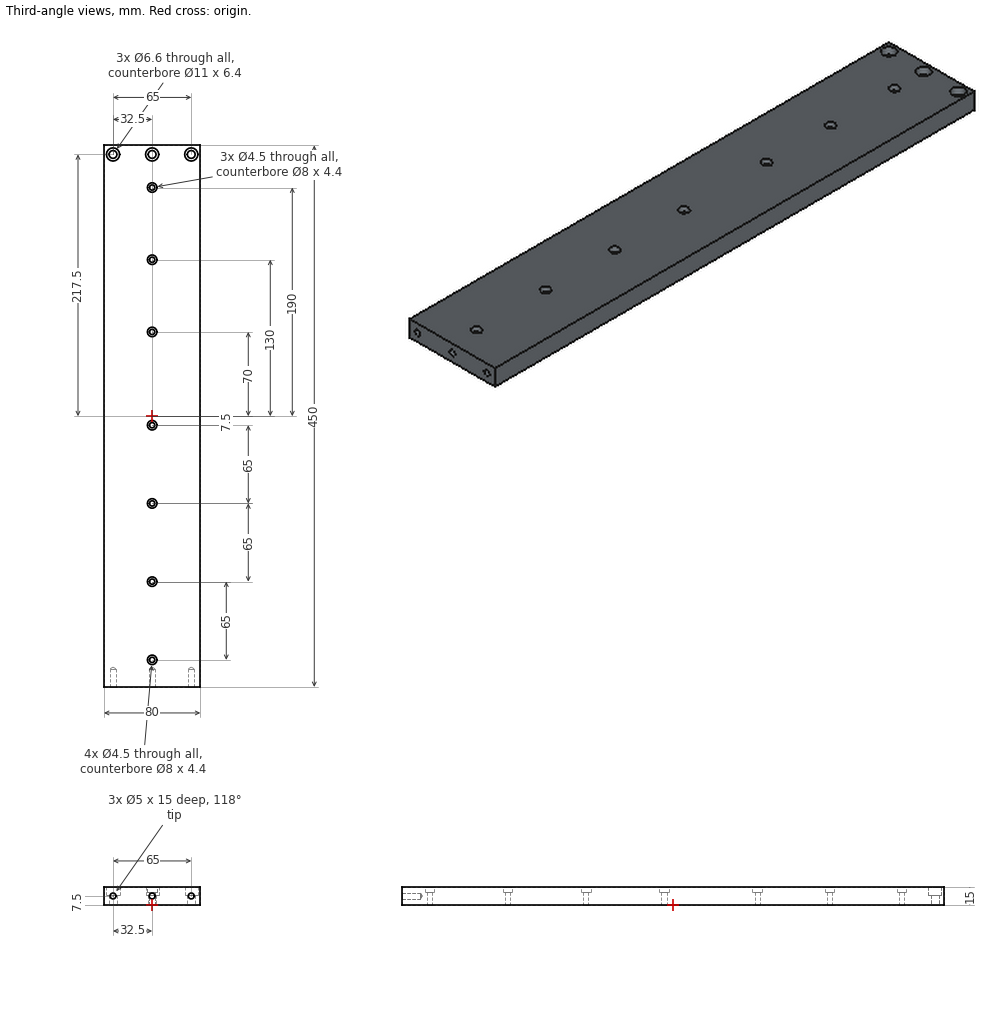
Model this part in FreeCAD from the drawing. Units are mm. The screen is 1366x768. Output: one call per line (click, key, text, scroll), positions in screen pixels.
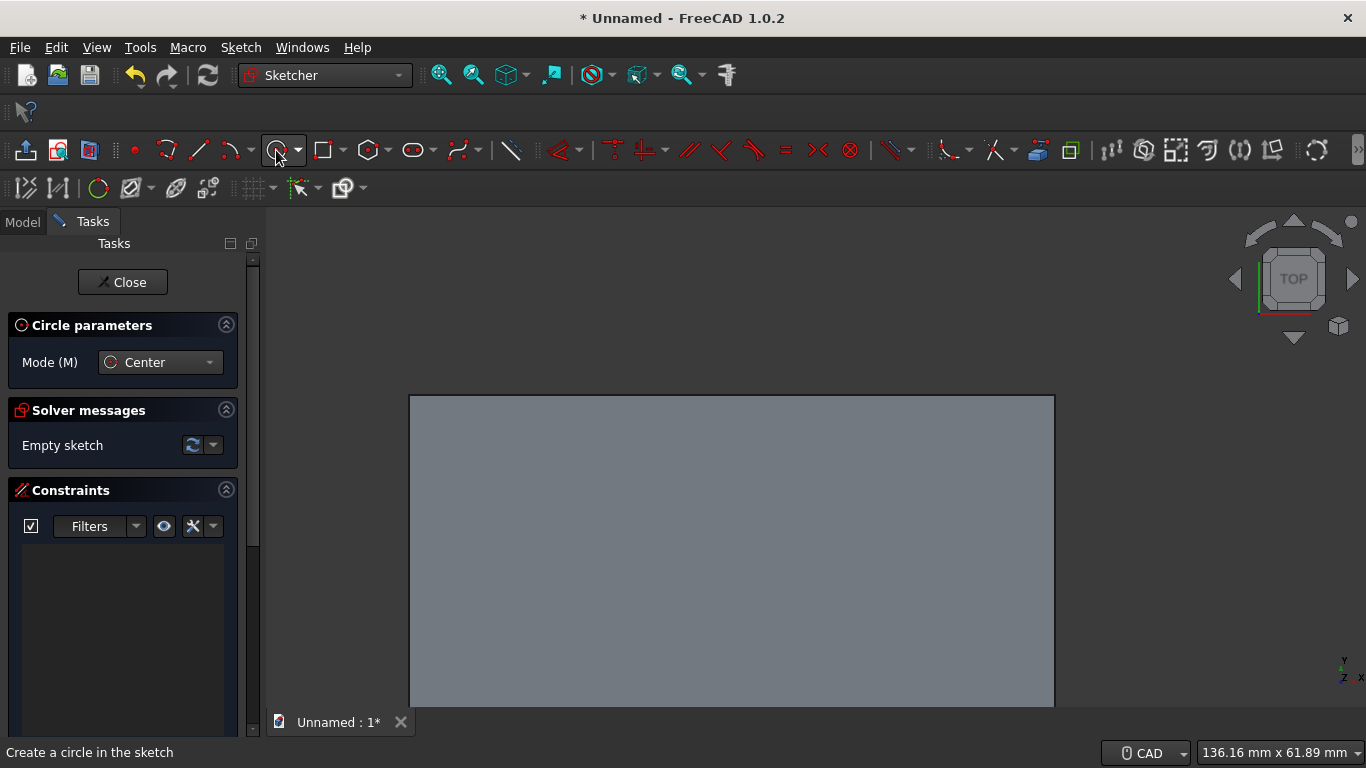
click(469, 456)
move(488, 437)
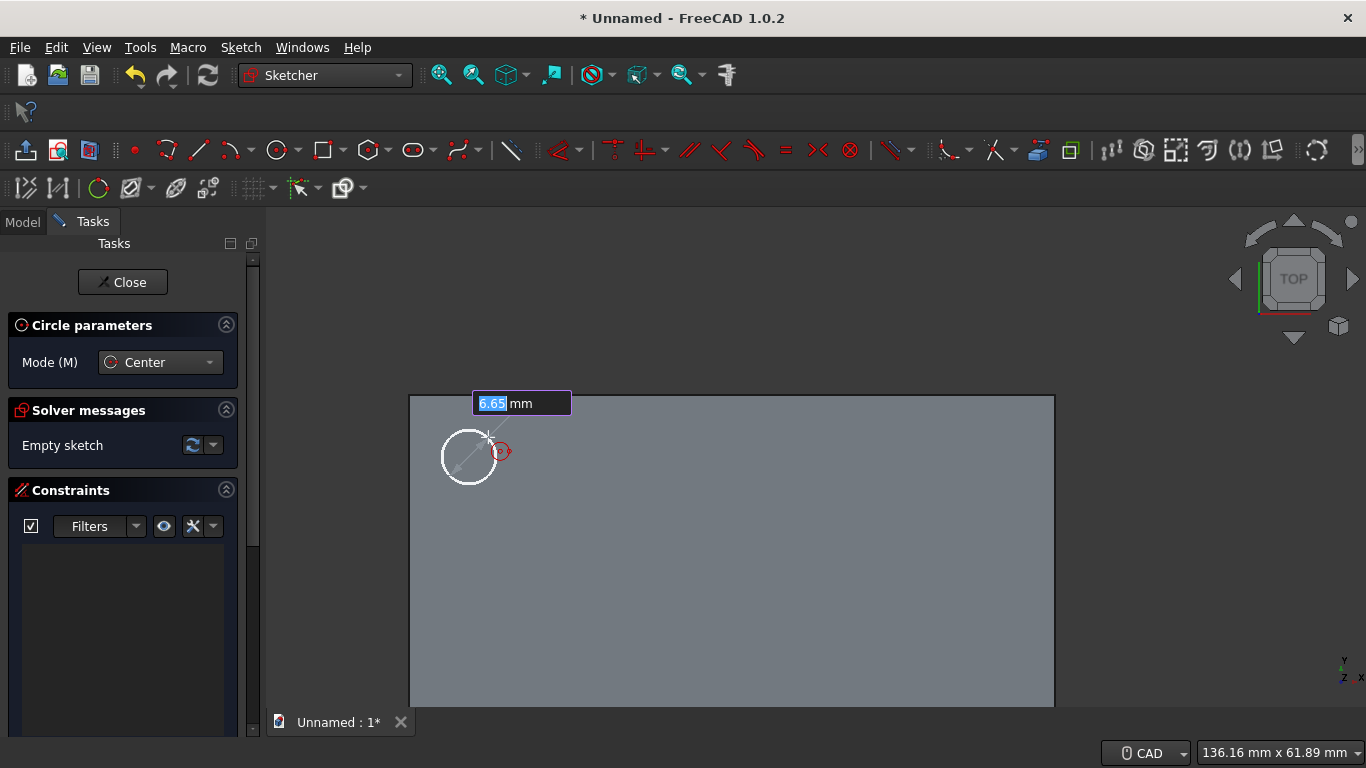
text(6.6)
key(Return)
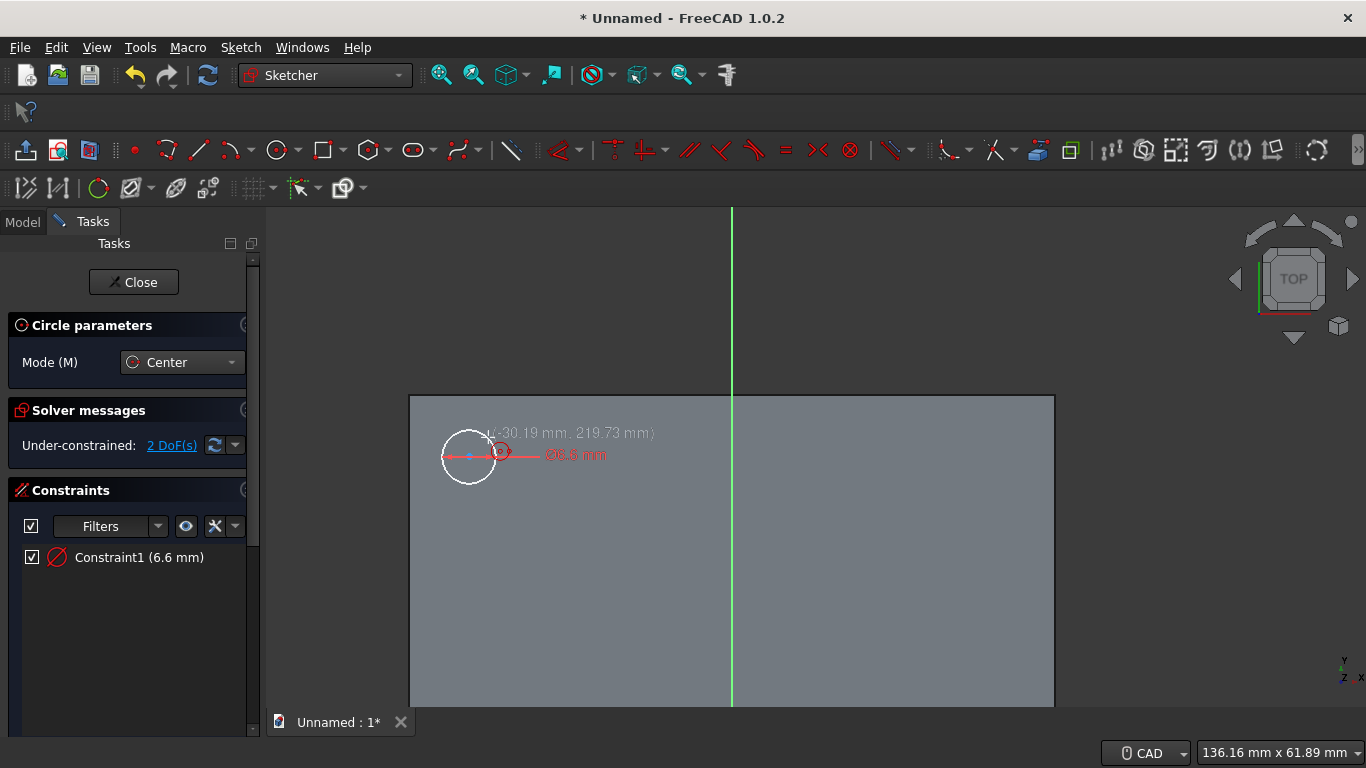
click(994, 456)
move(1013, 437)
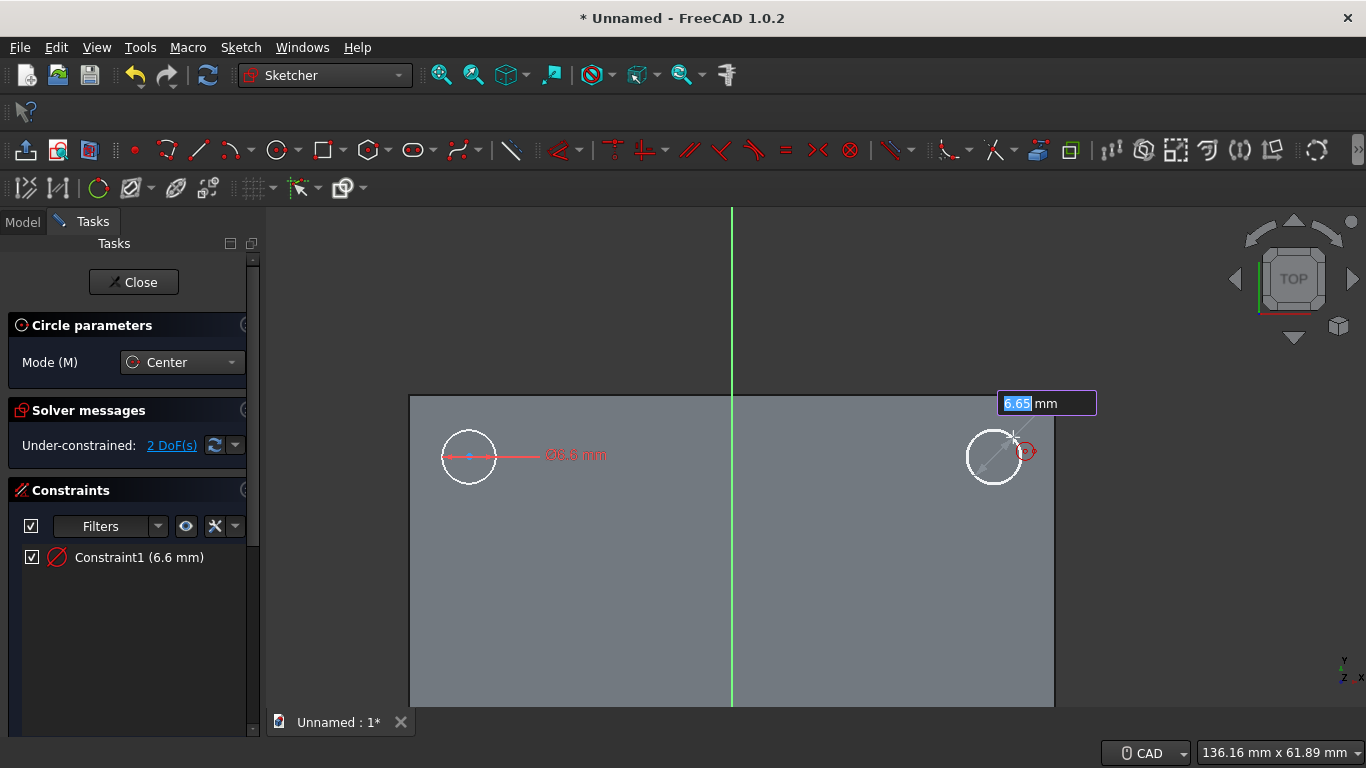
text(6.6)
key(Return)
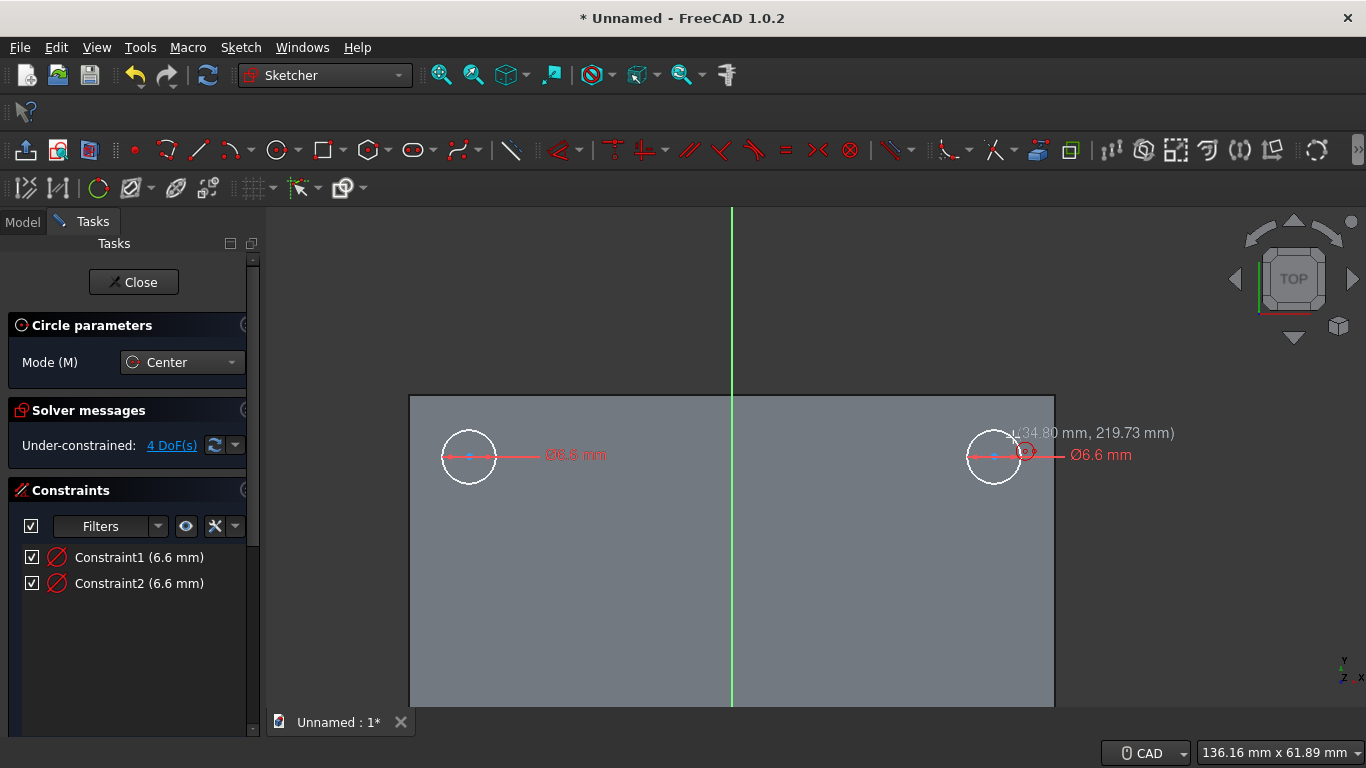
click(732, 456)
move(751, 437)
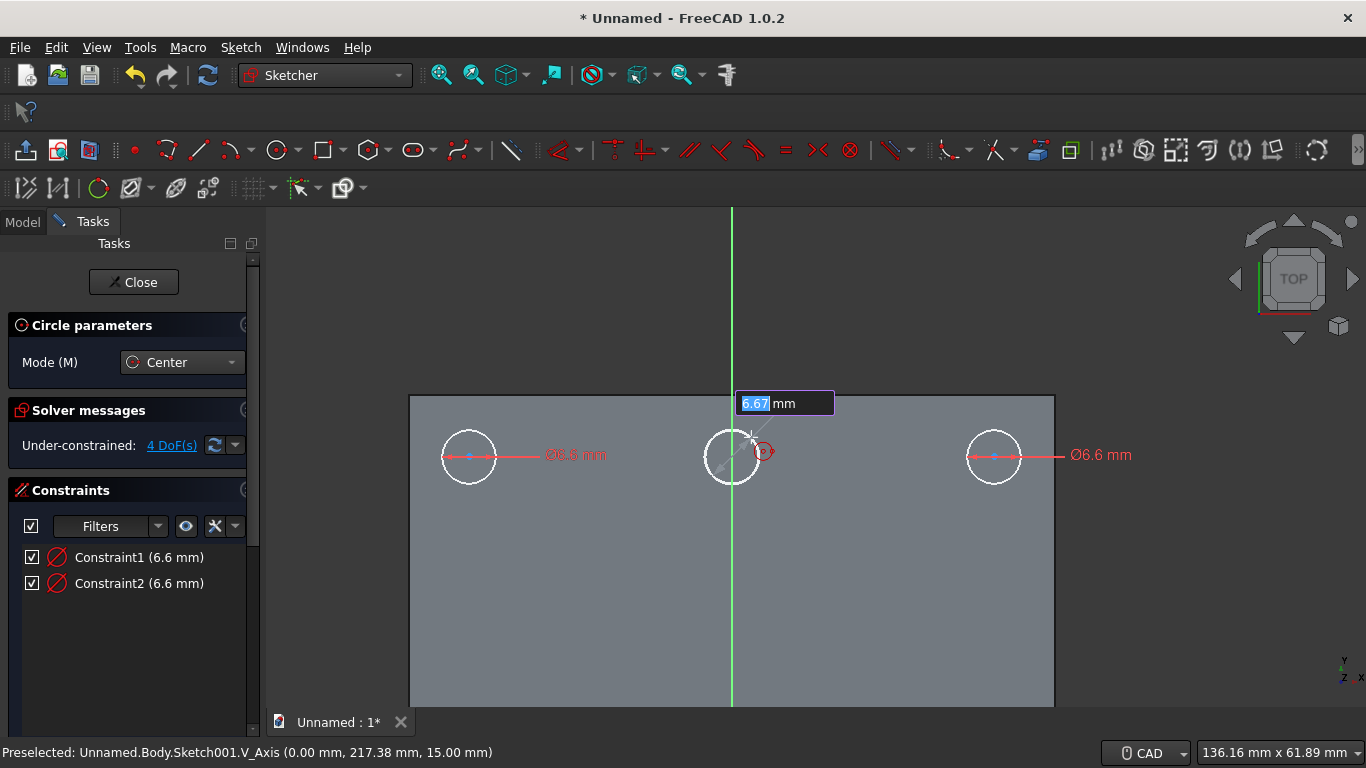
text(6.6)
key(Return)
key(Escape)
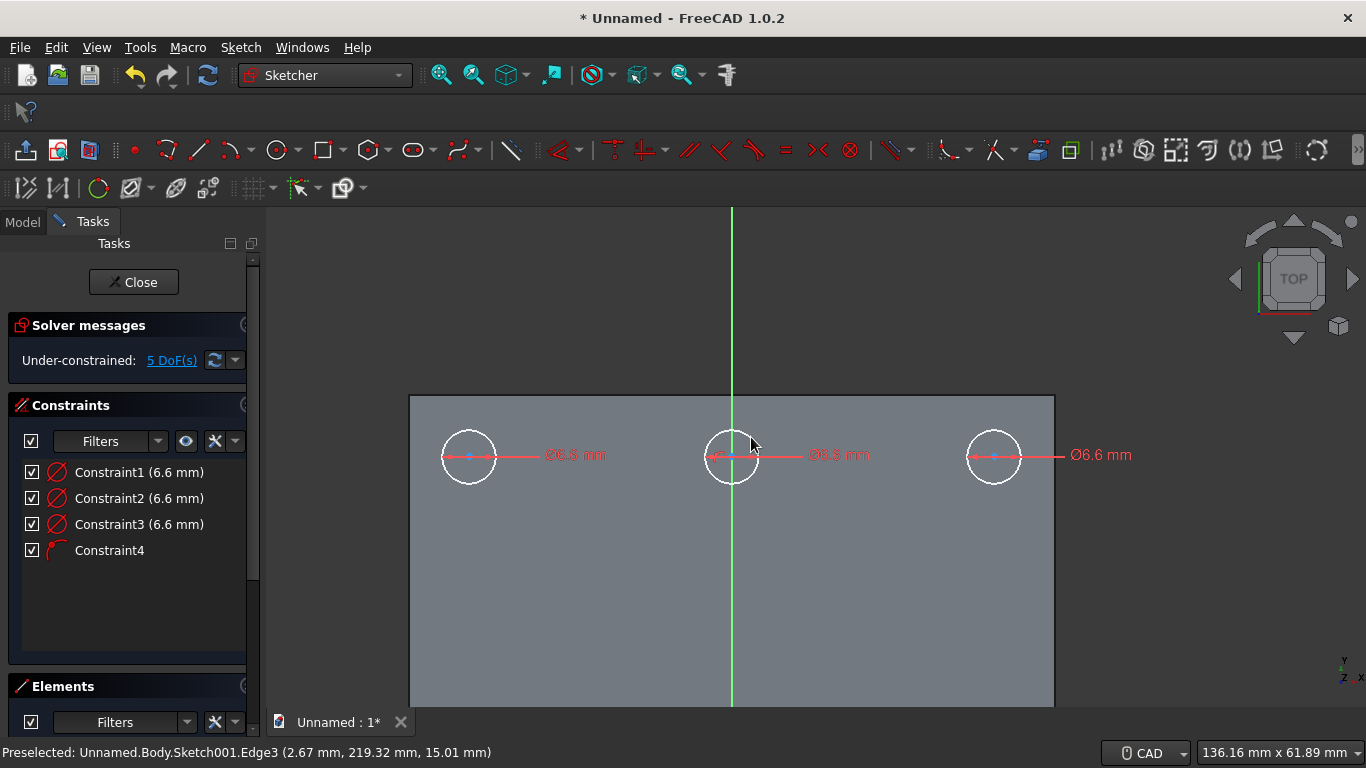
click(469, 457)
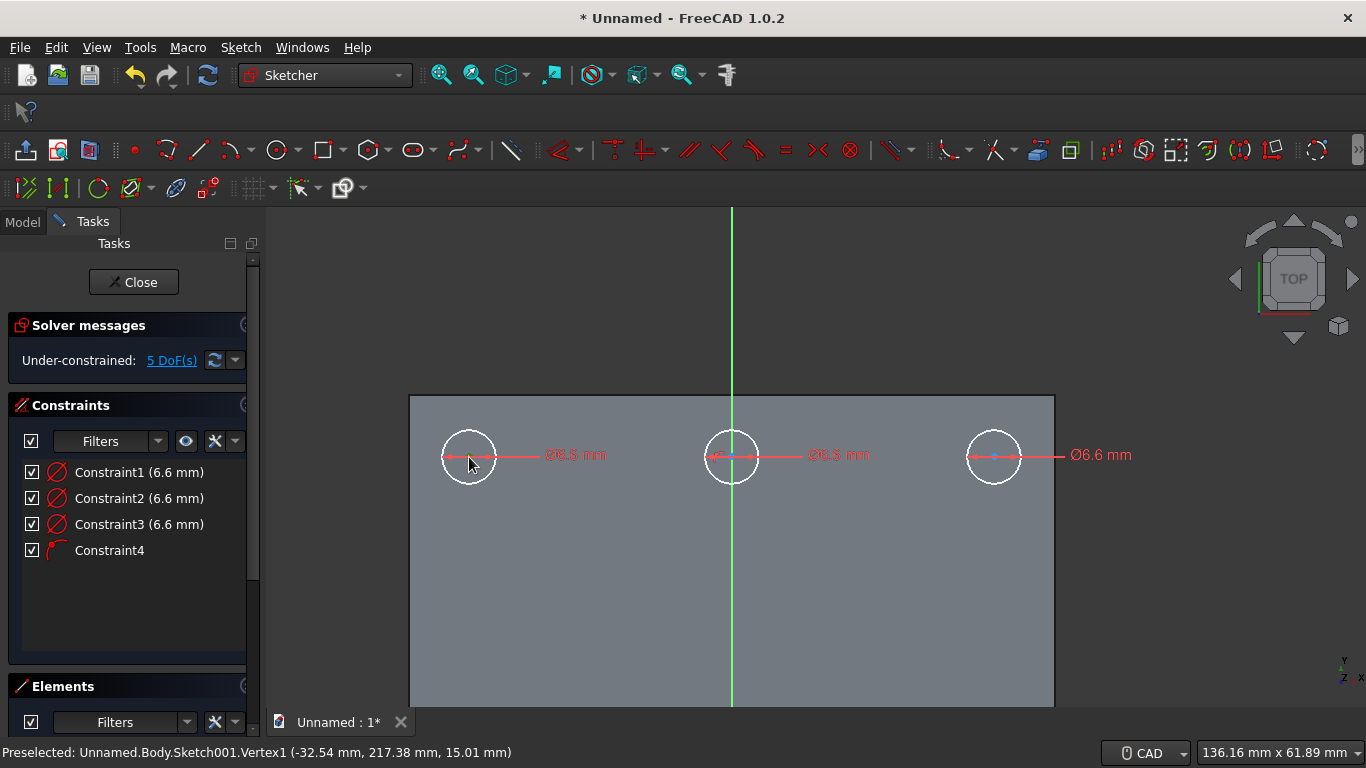
click(994, 457)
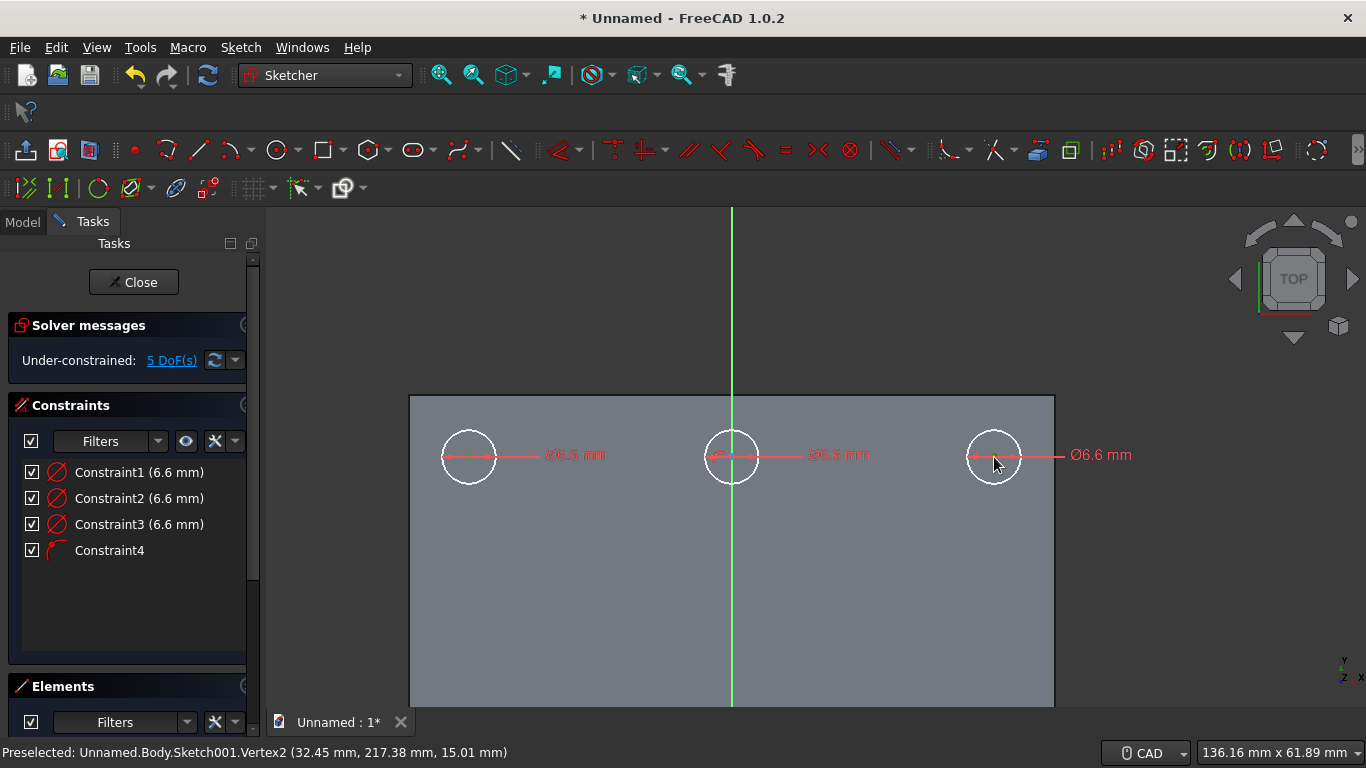
click(668, 150)